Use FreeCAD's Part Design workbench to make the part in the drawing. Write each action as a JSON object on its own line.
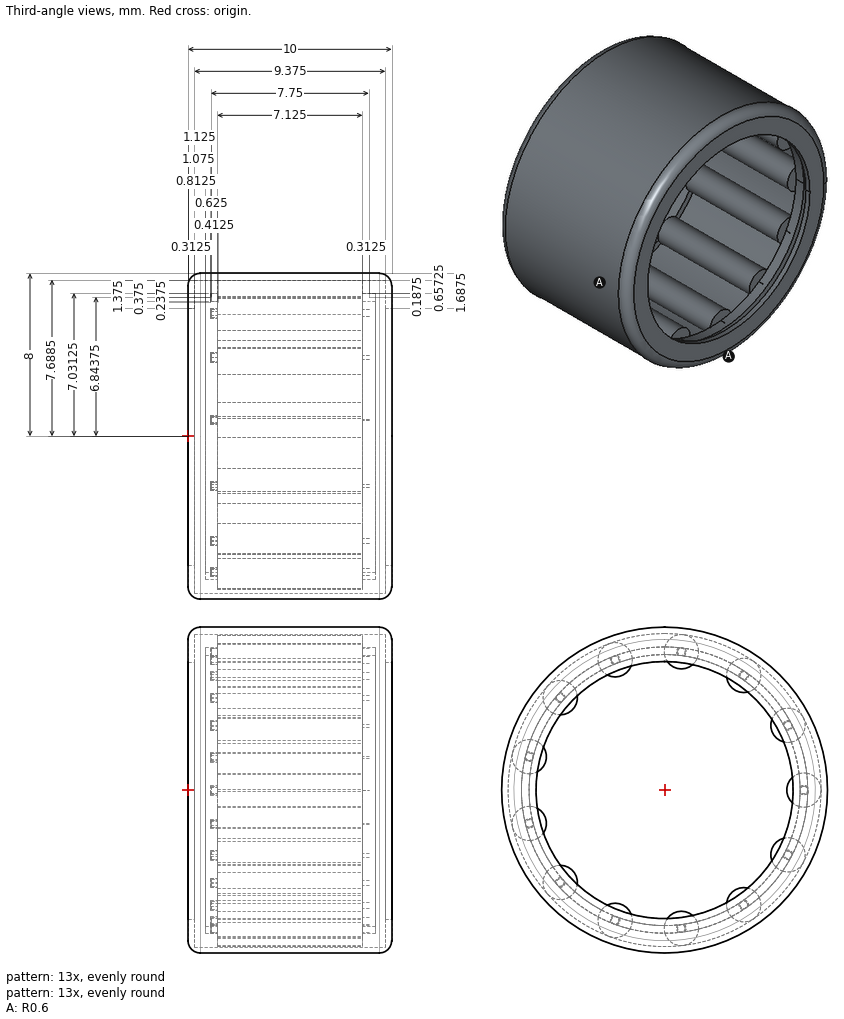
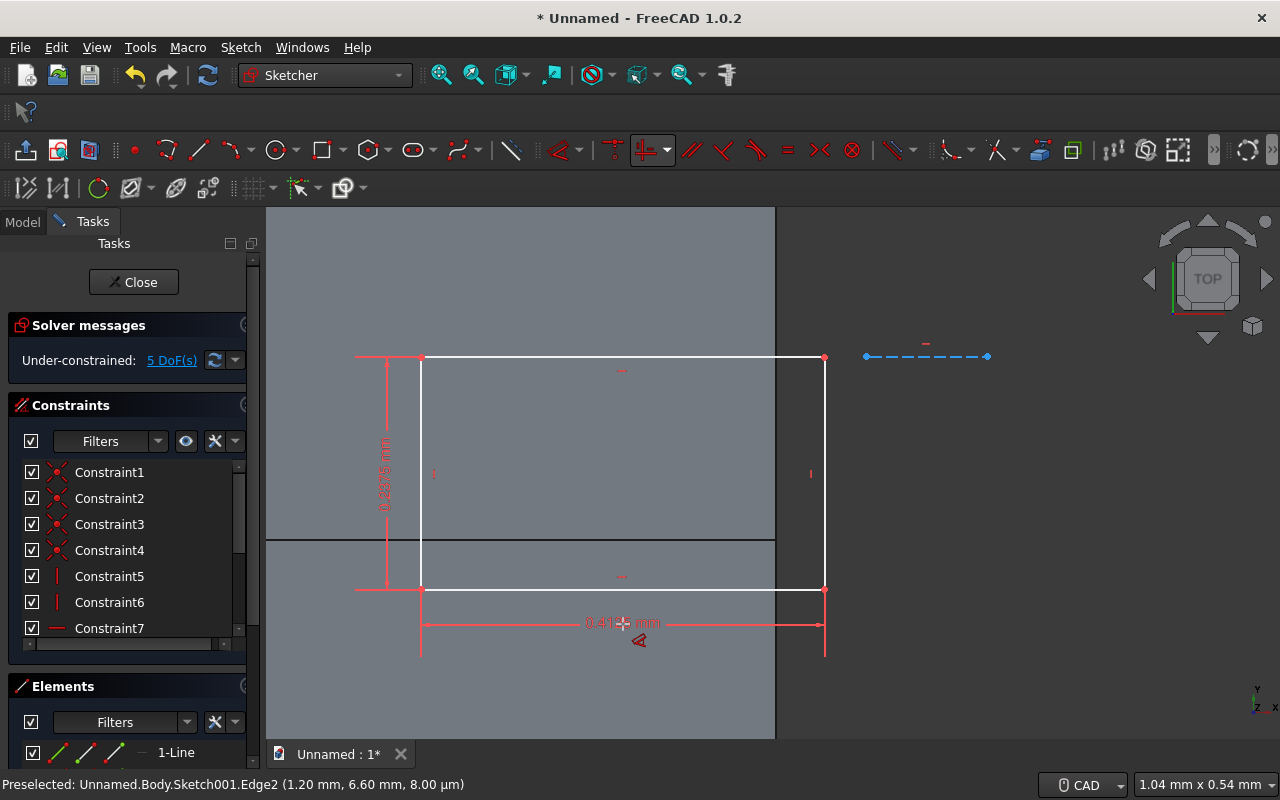
{"action": "left_click", "coordinate": [421, 357]}
{"action": "left_click", "coordinate": [357, 323]}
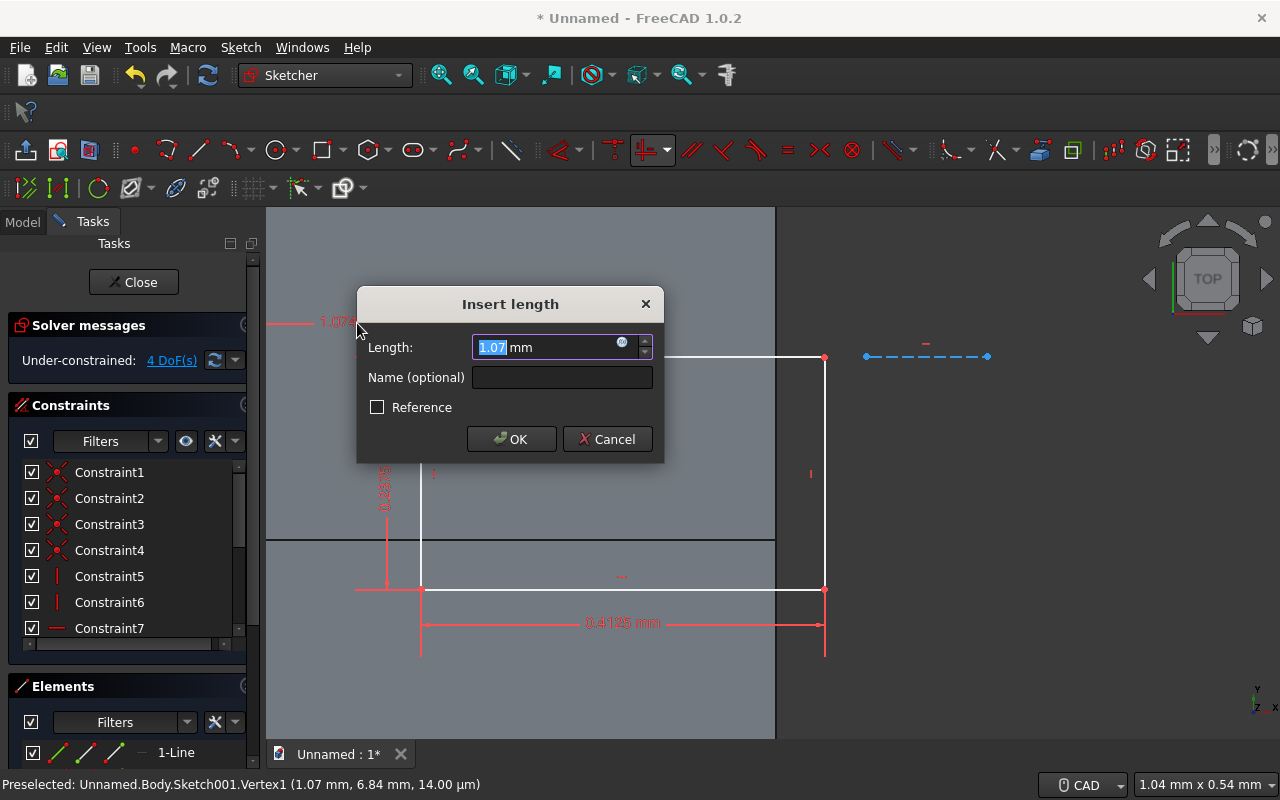
{"action": "type", "text": "1.075"}
{"action": "key", "text": "Return"}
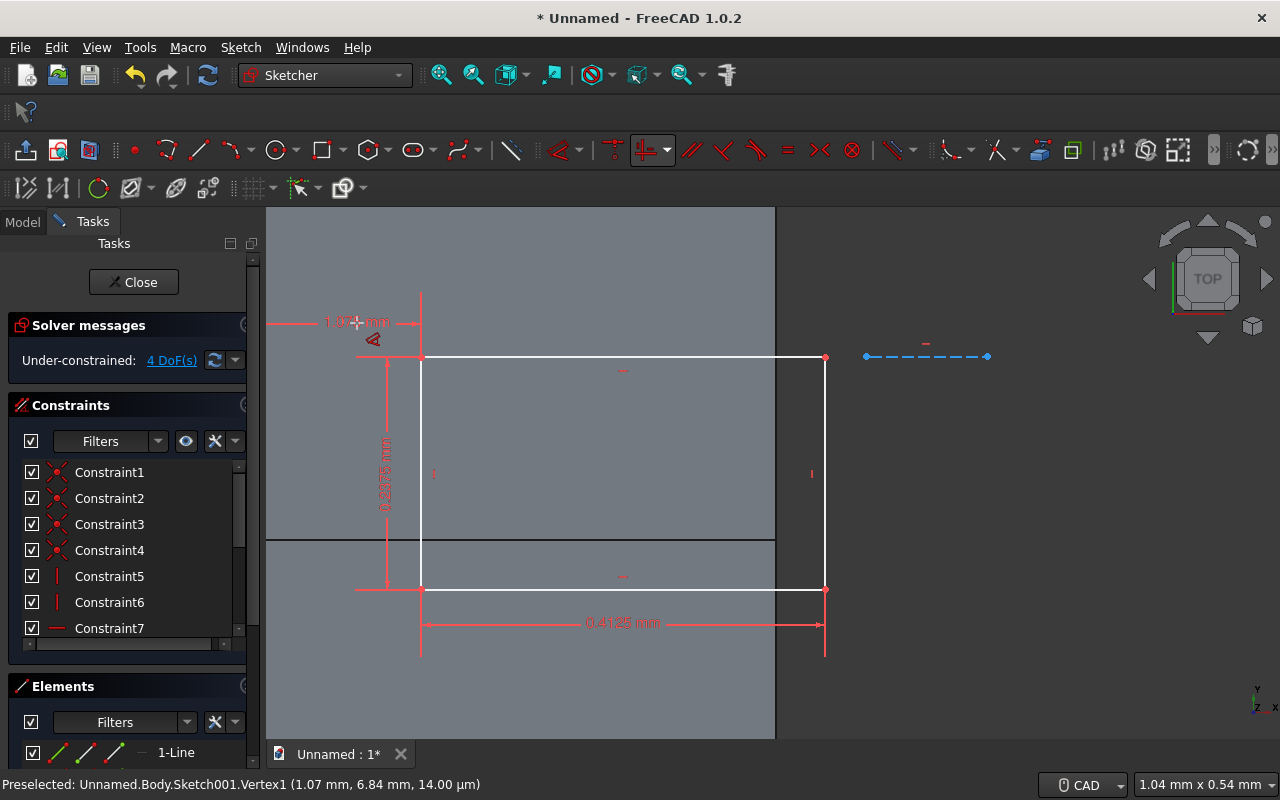
{"action": "left_click", "coordinate": [421, 357]}
{"action": "left_click", "coordinate": [455, 534]}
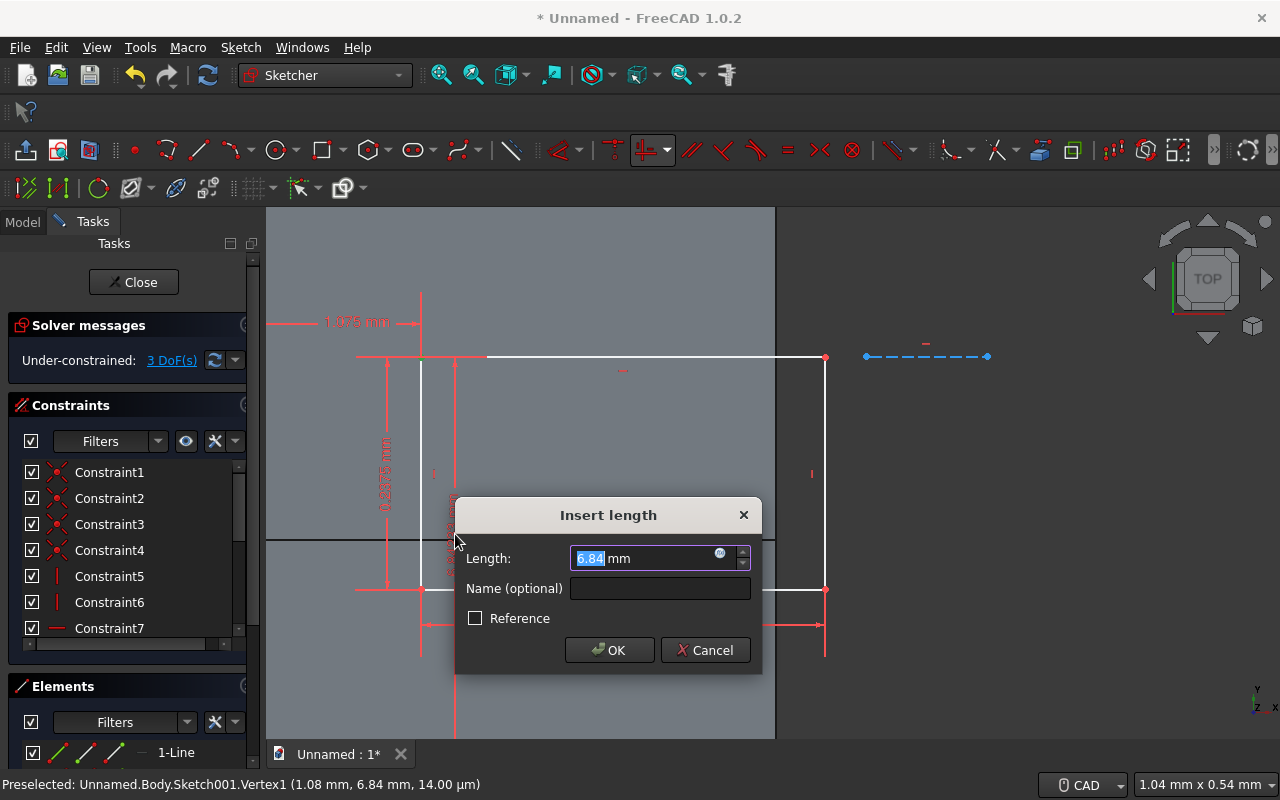
{"action": "type", "text": "6.84375"}
{"action": "key", "text": "Return"}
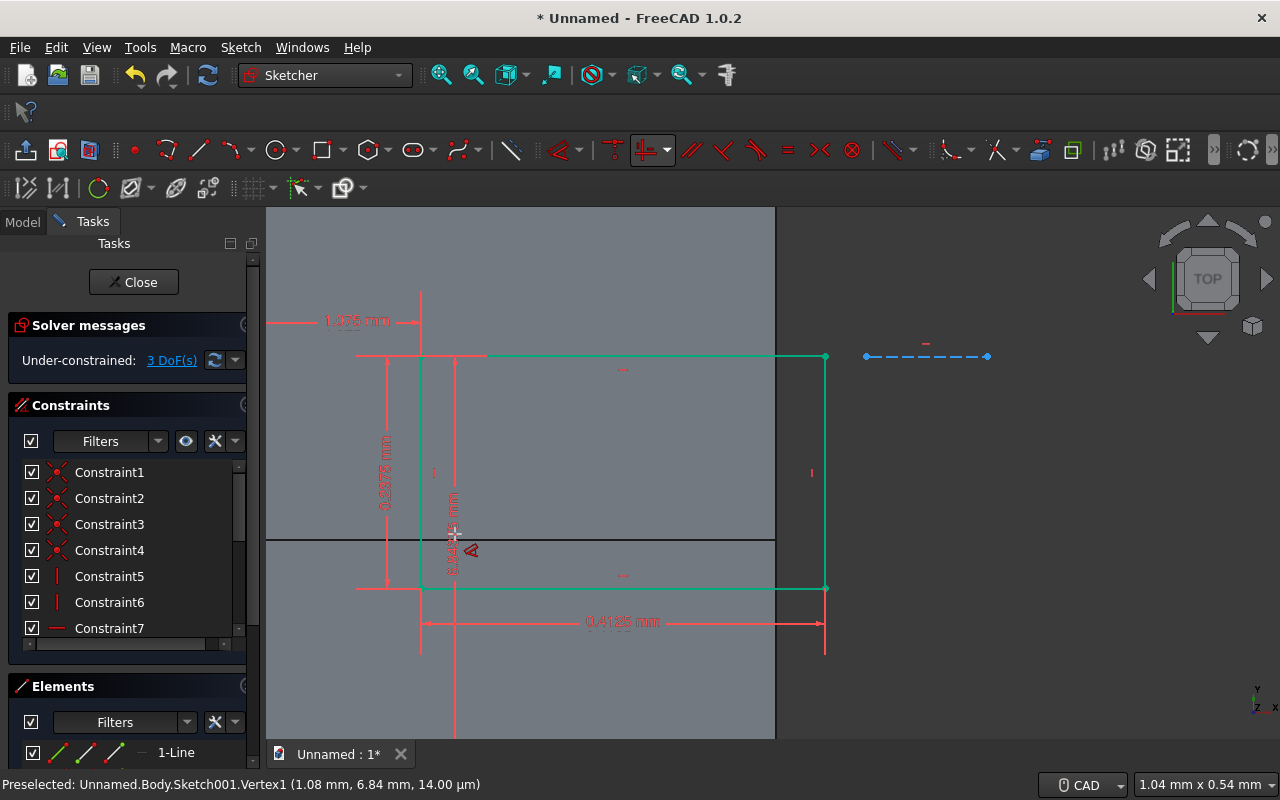
{"action": "left_click", "coordinate": [866, 357]}
{"action": "left_click", "coordinate": [900, 534]}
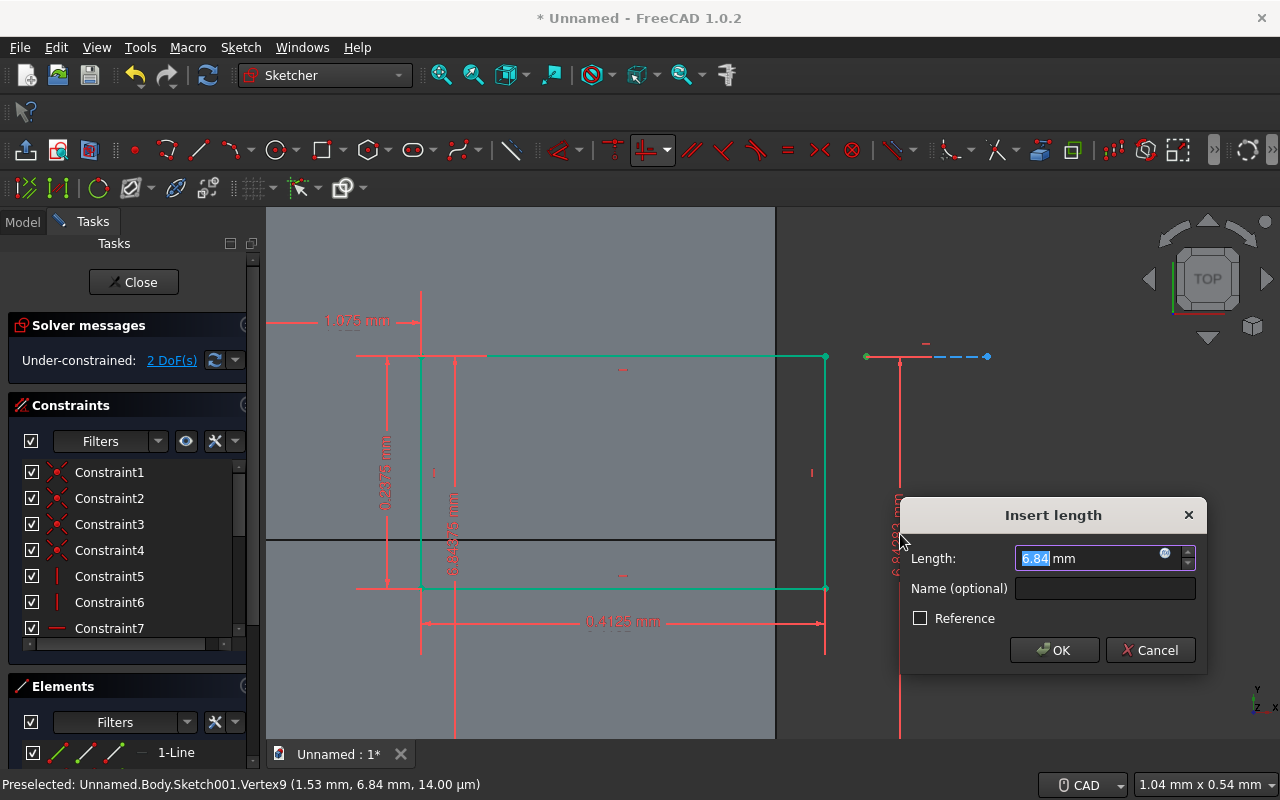
{"action": "type", "text": "6.84375"}
{"action": "key", "text": "Return"}
{"action": "key", "text": "Escape"}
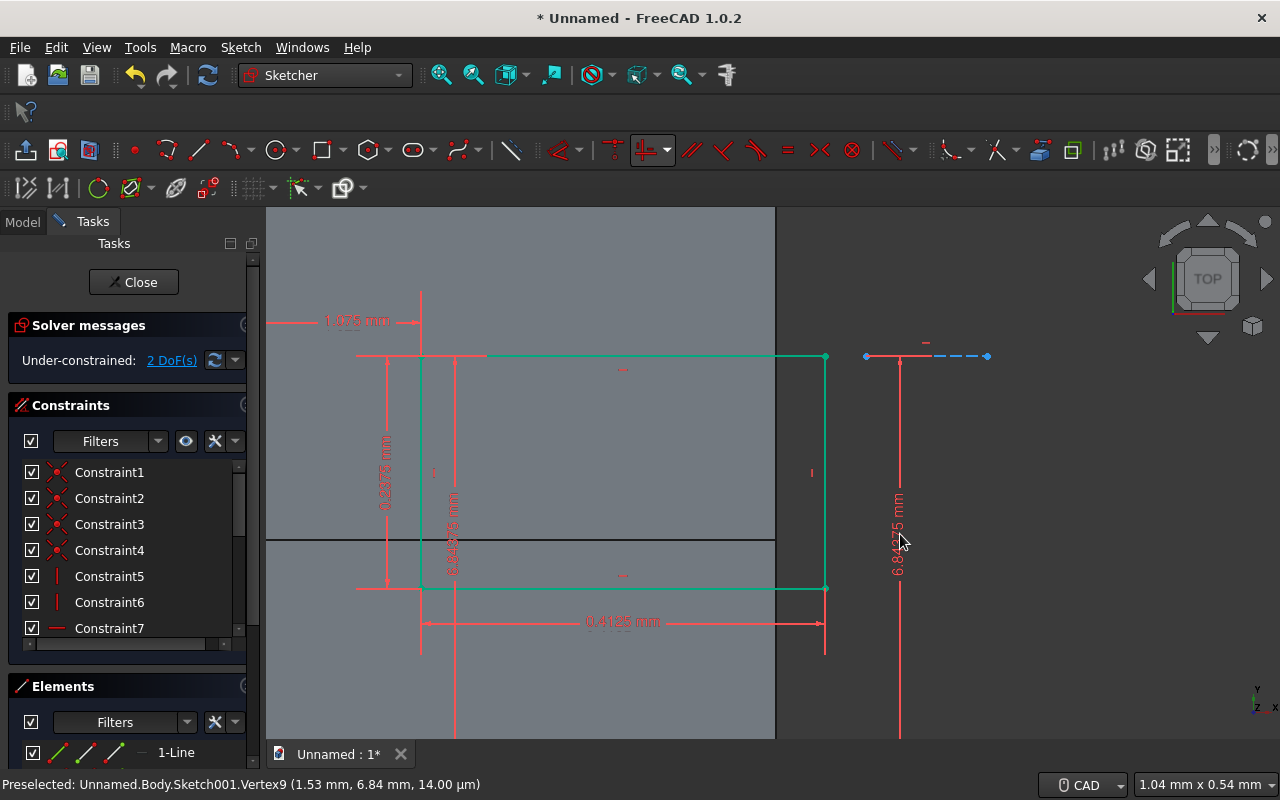
{"action": "left_click", "coordinate": [134, 282]}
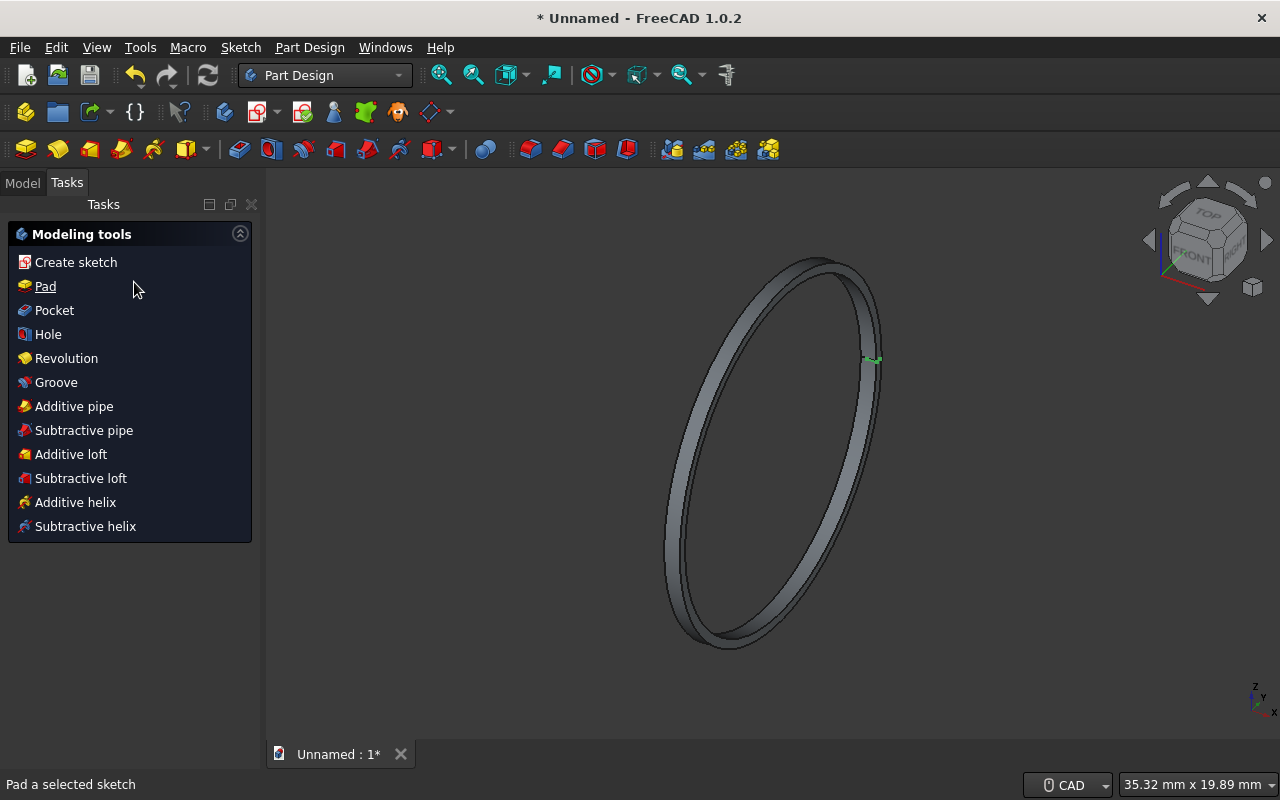
{"action": "left_click", "coordinate": [304, 150]}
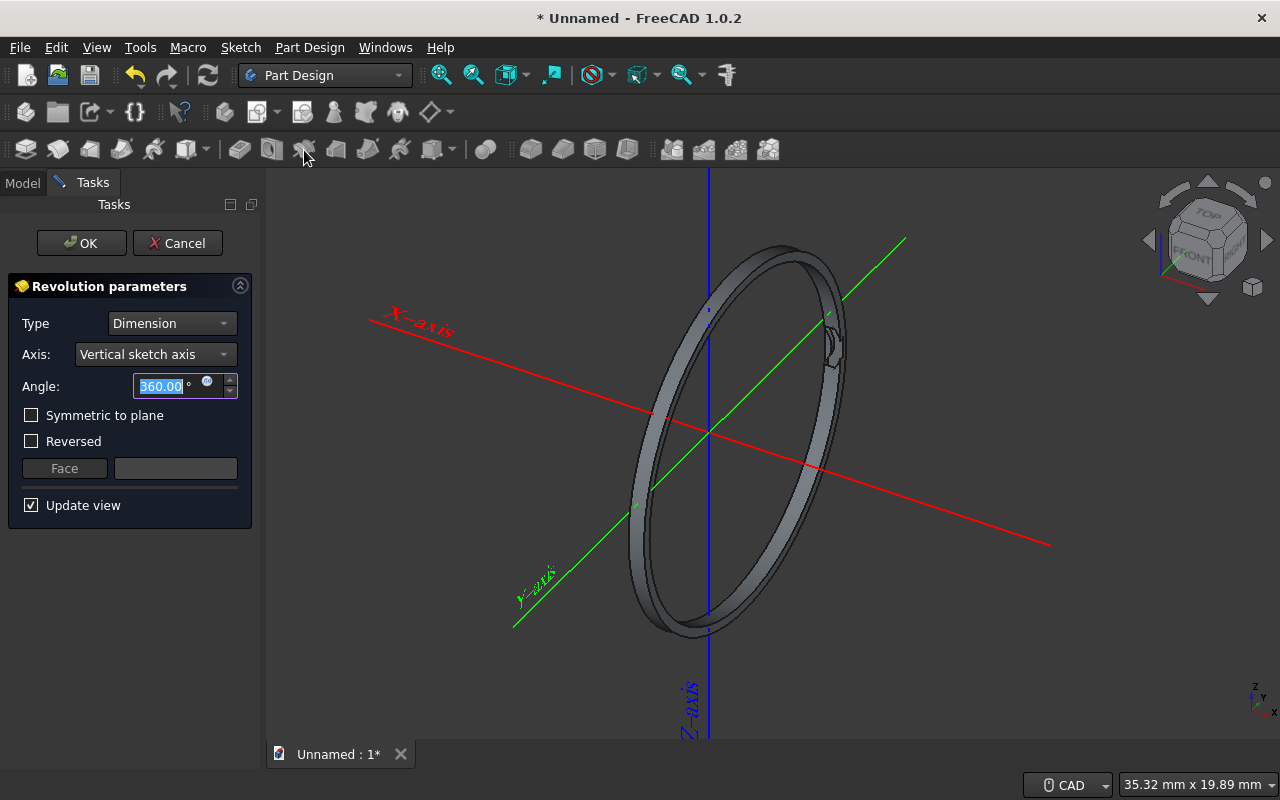
{"action": "left_click", "coordinate": [156, 354]}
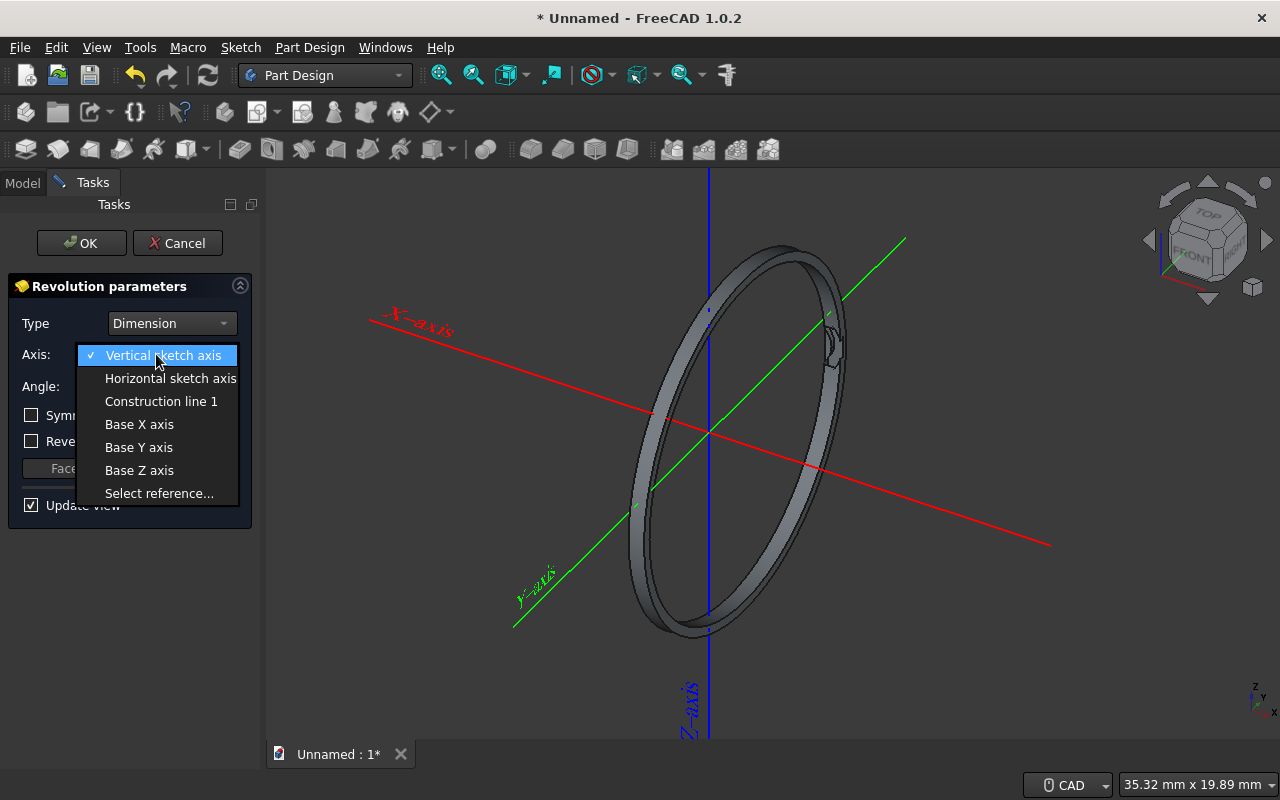
{"action": "left_click", "coordinate": [156, 402]}